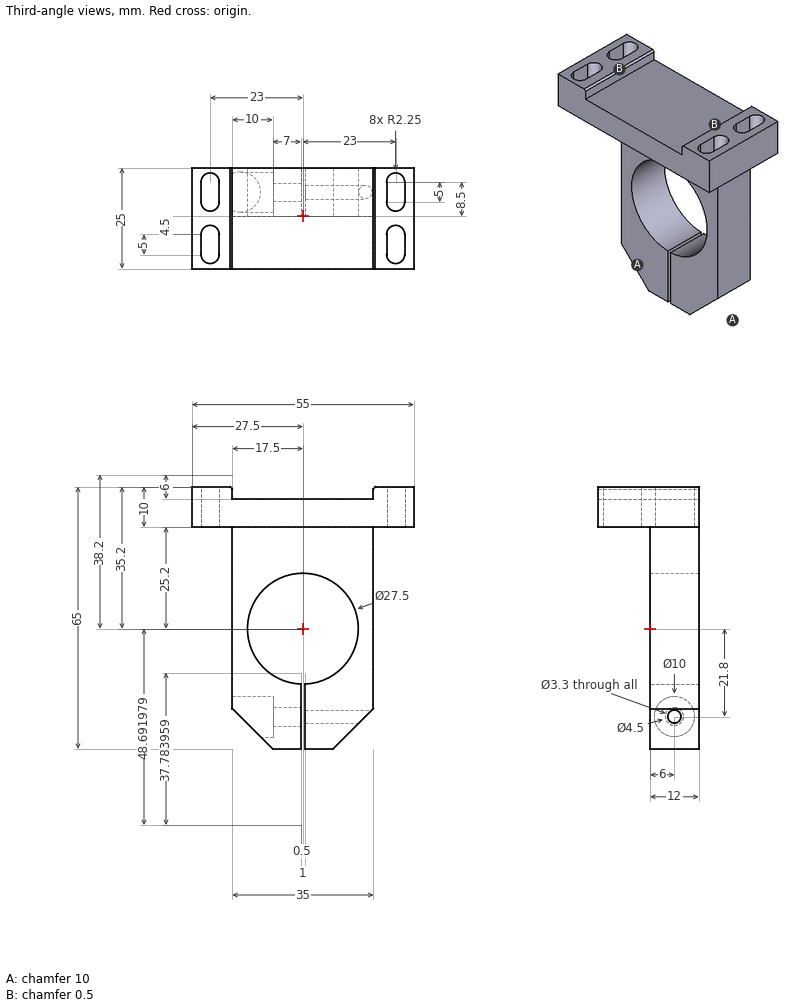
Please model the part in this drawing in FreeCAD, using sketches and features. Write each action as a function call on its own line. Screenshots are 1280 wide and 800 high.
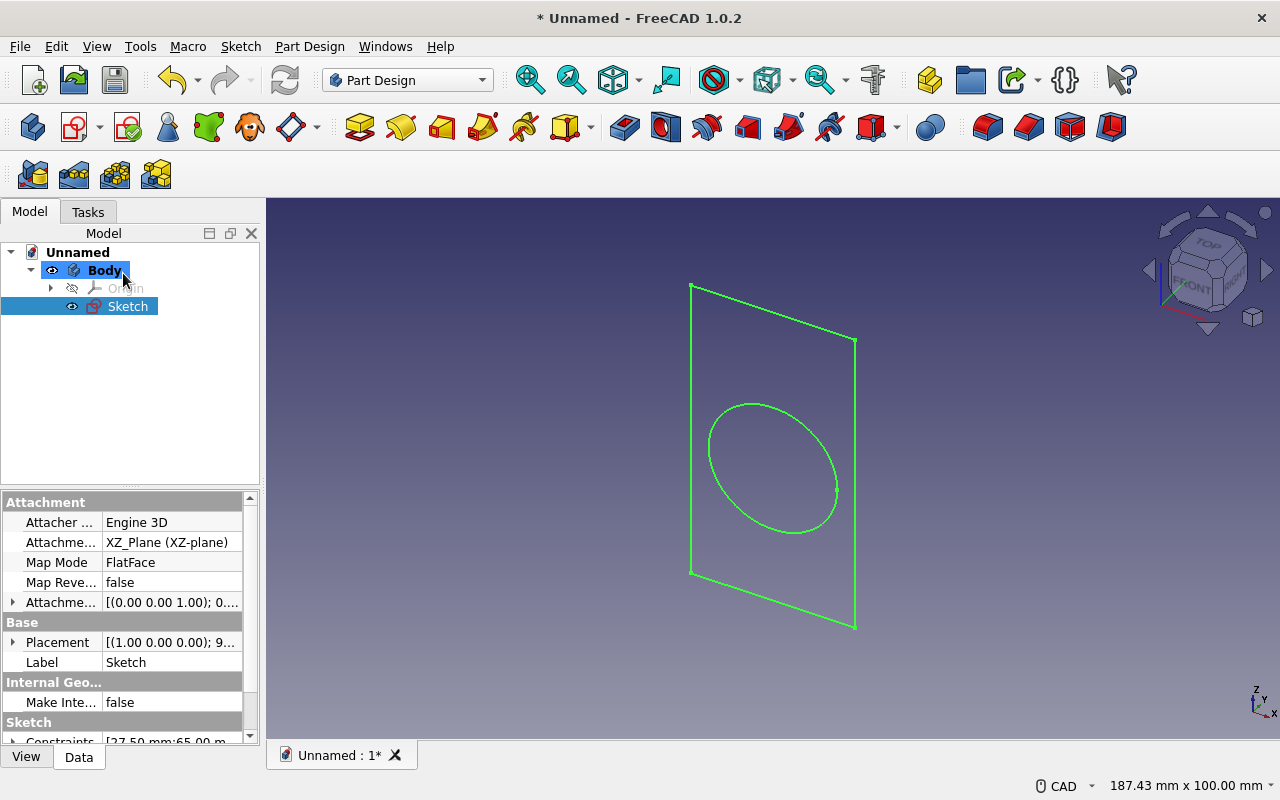
click(360, 128)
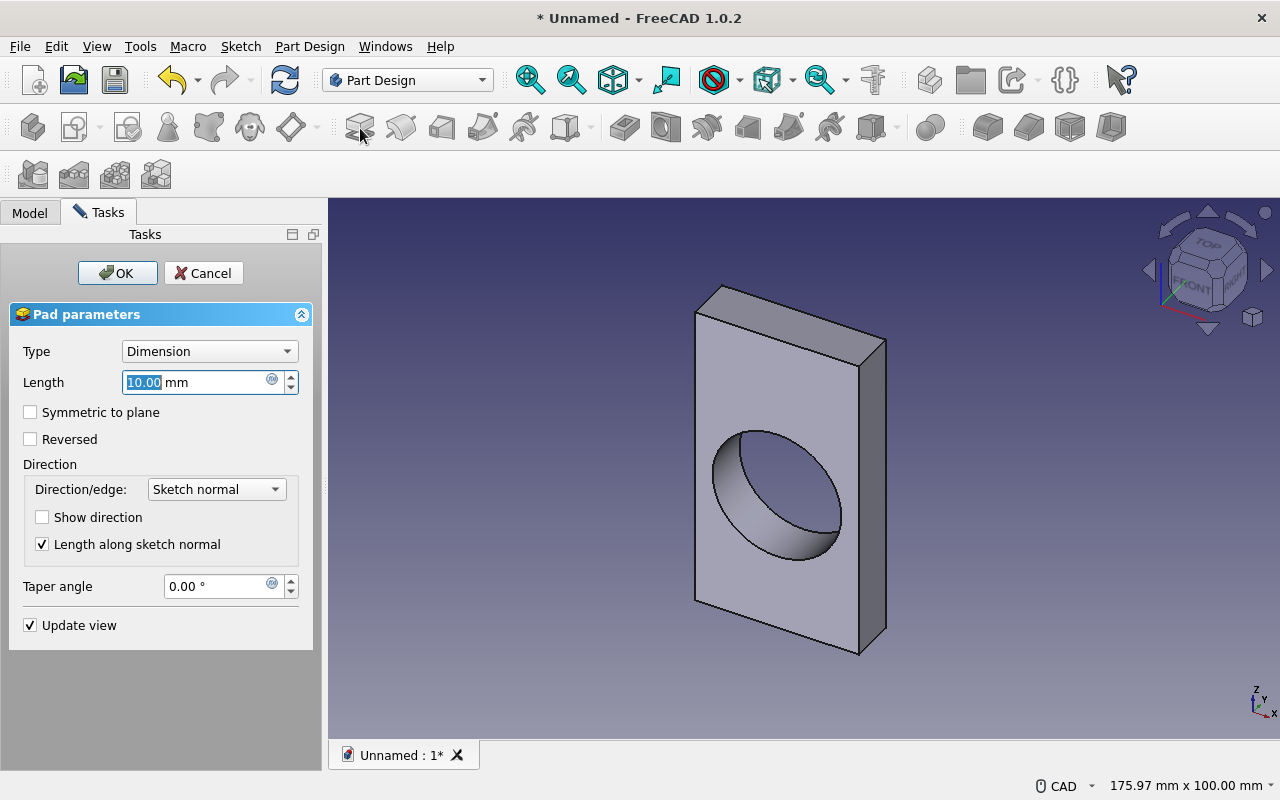
text(12)
key(Tab)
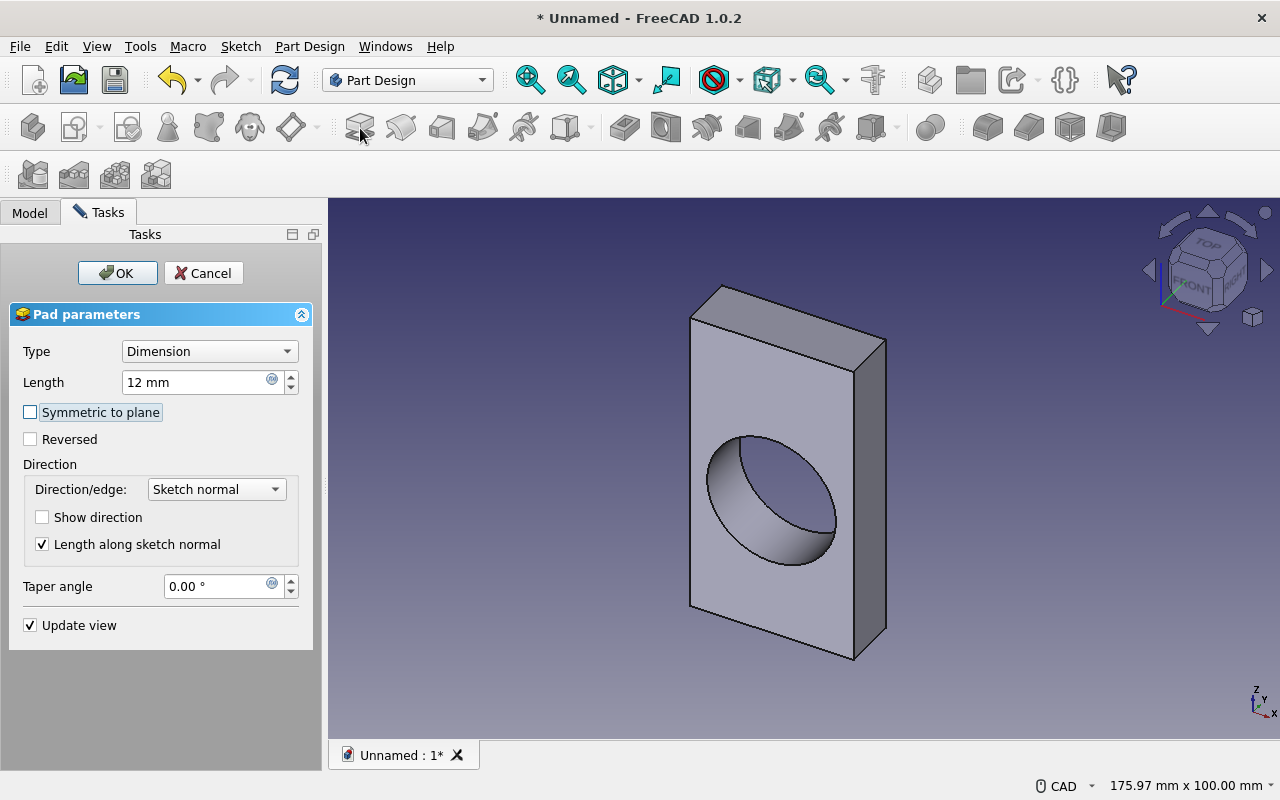
click(31, 439)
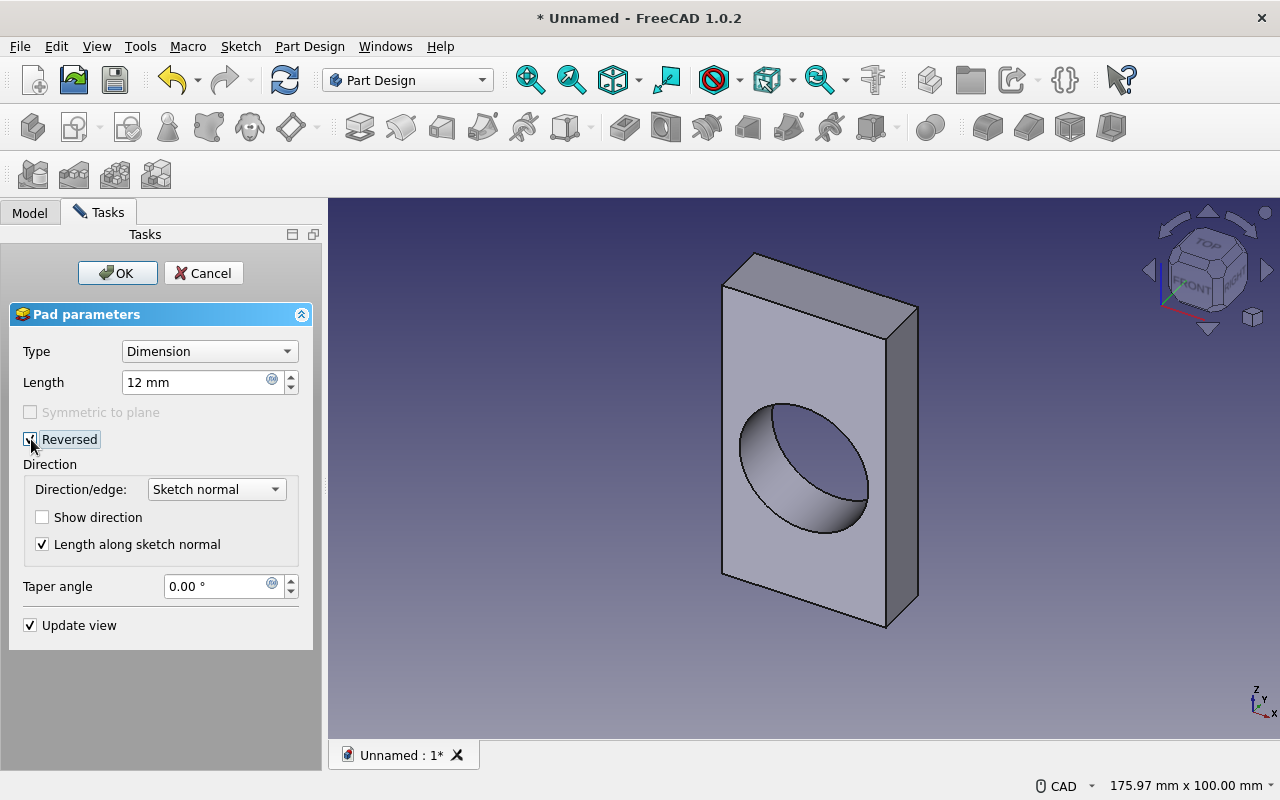
click(118, 273)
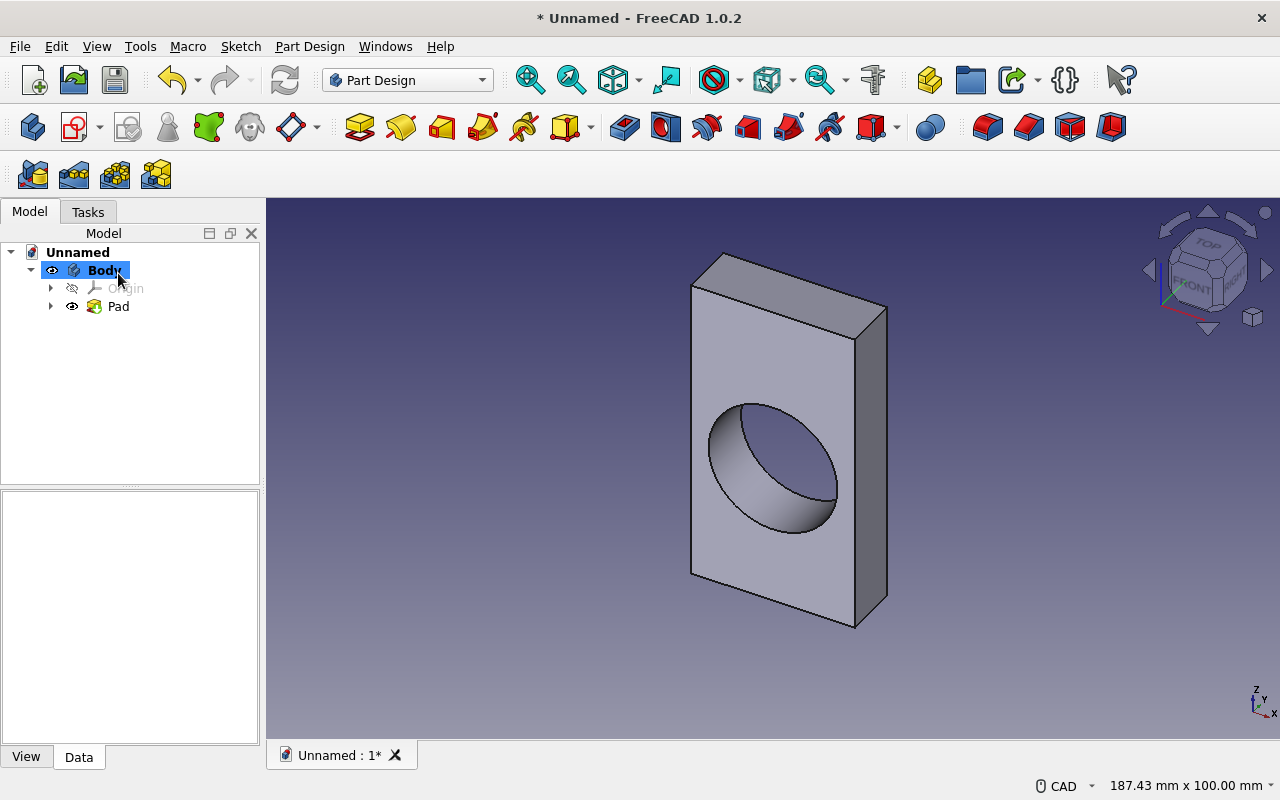
key(0)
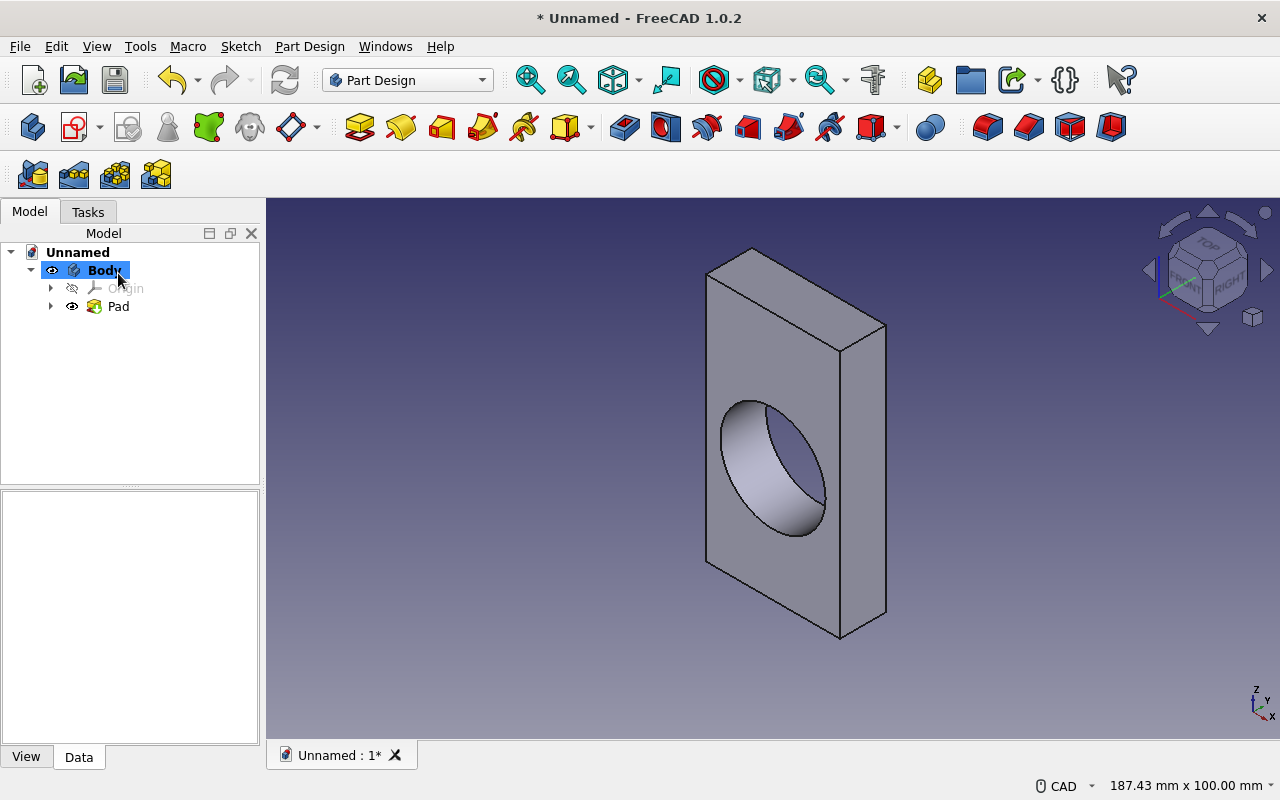
key(2)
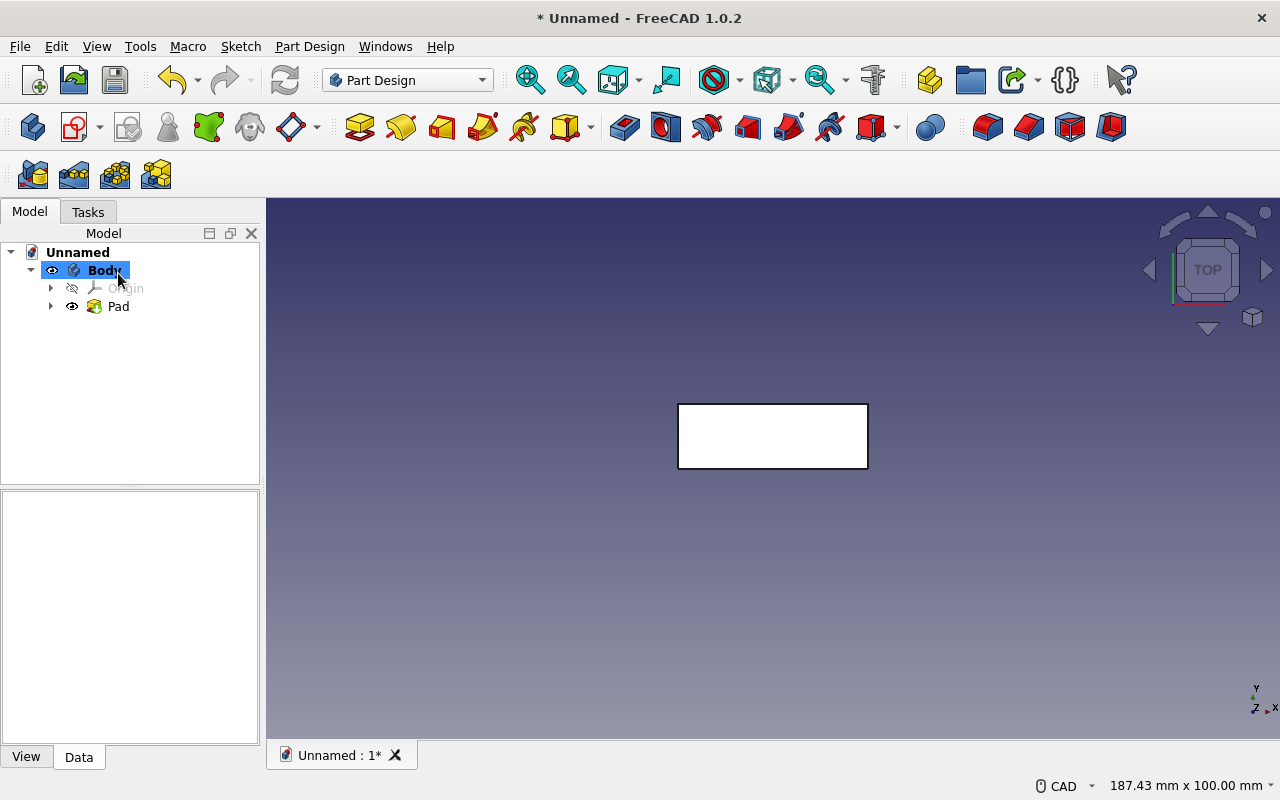
key(v)
key(f)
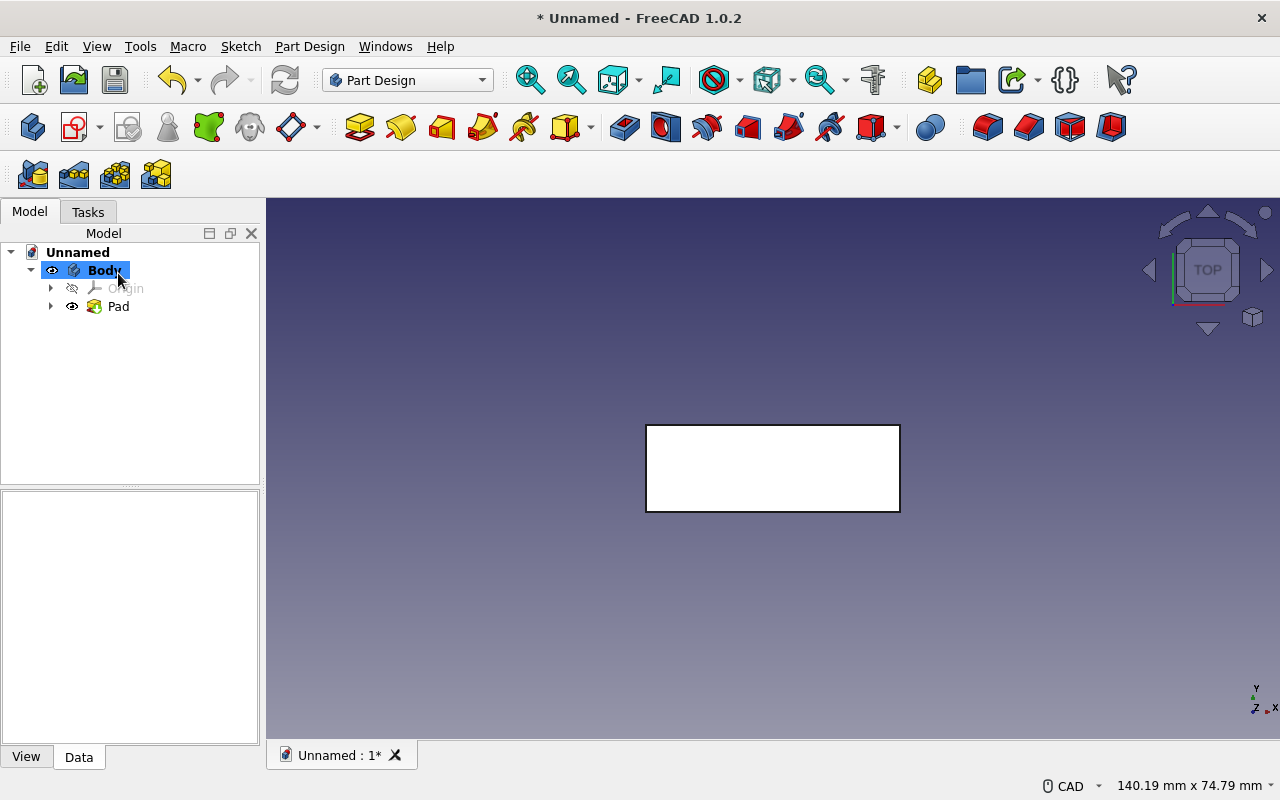
key(1)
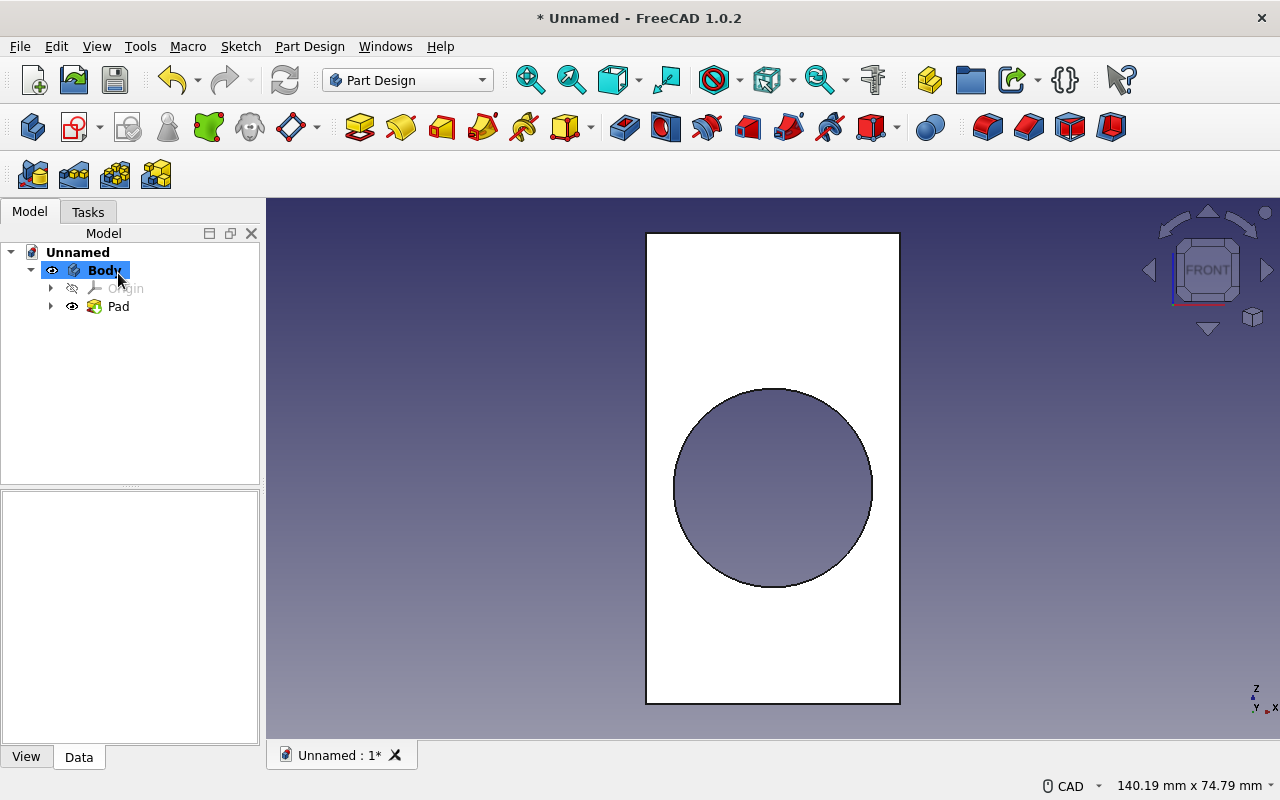
key(3)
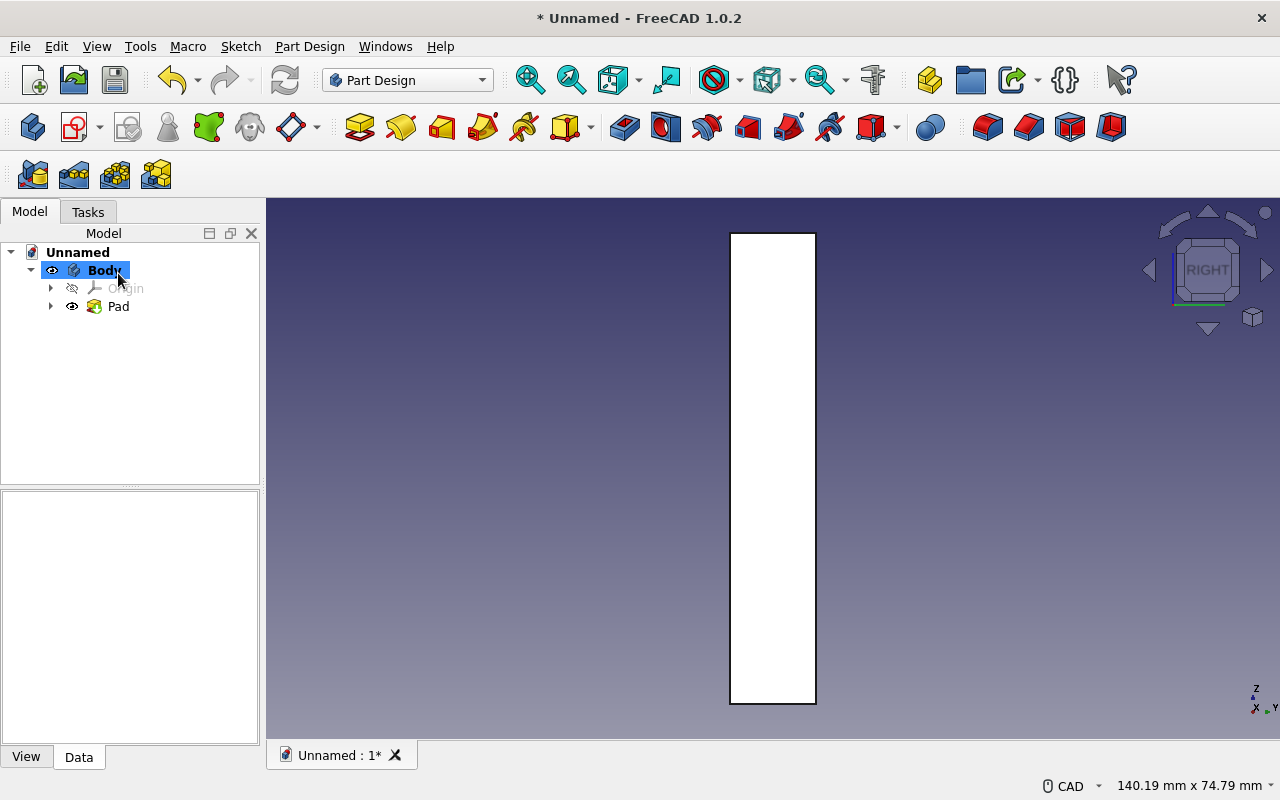
click(773, 703)